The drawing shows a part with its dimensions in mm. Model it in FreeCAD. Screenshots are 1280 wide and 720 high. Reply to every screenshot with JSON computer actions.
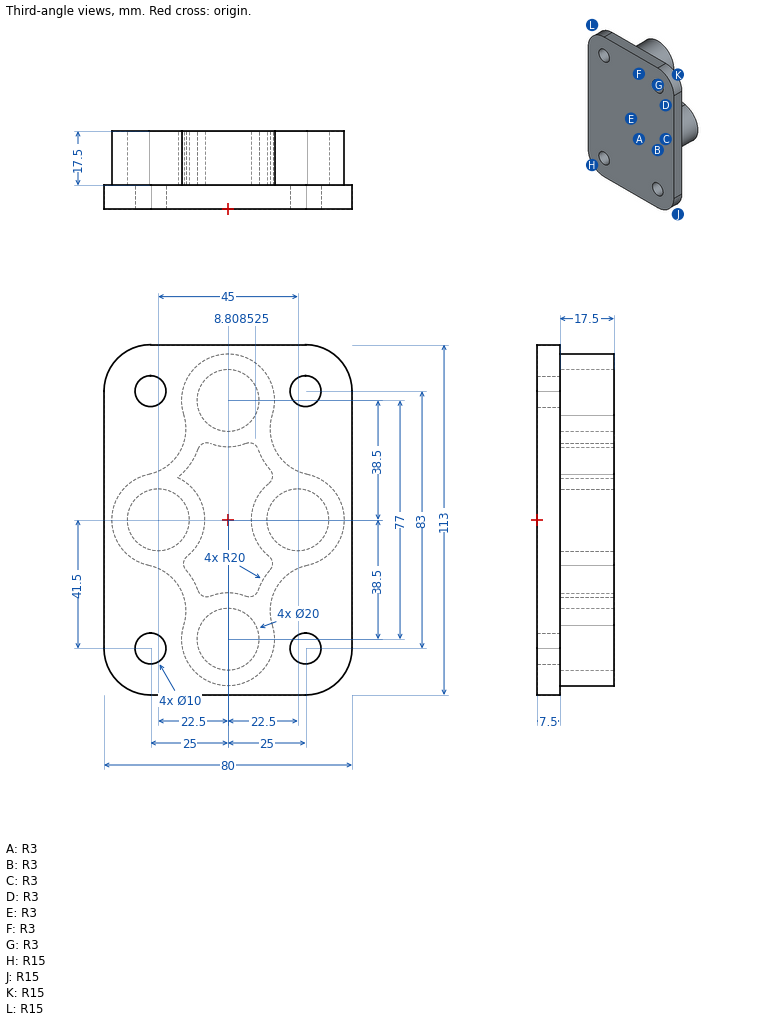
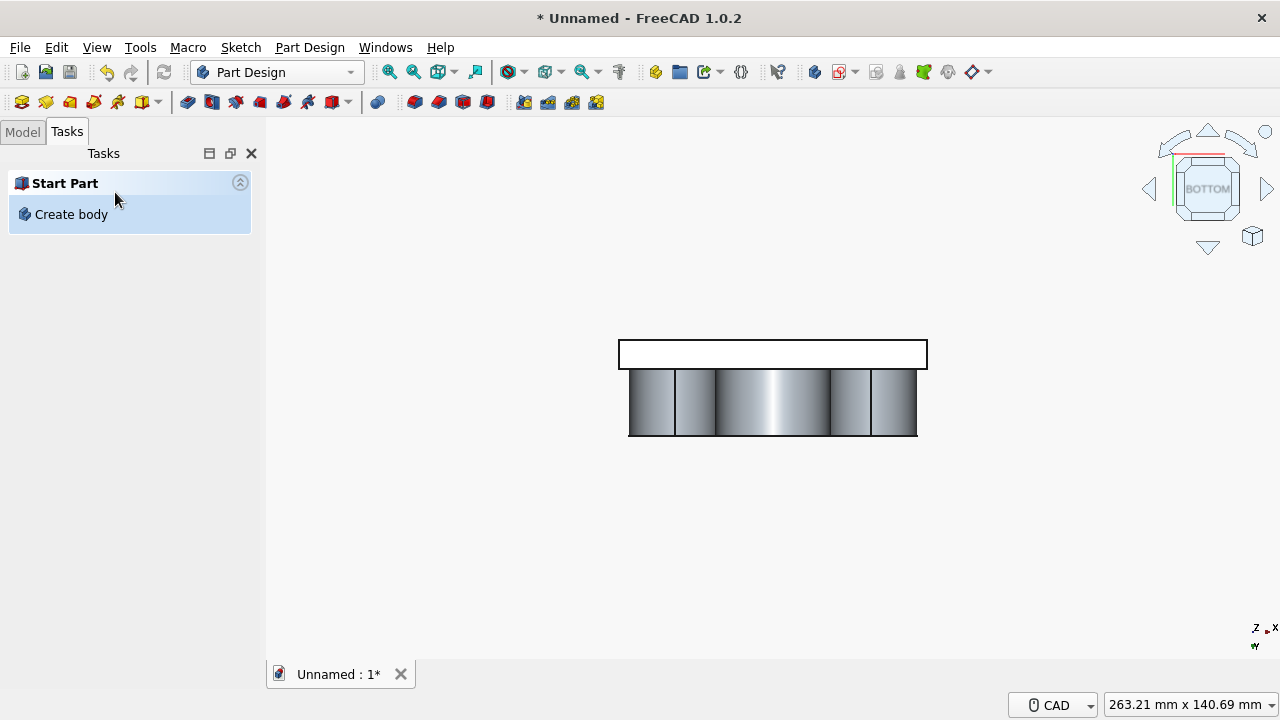
{"action": "left_click", "coordinate": [390, 72]}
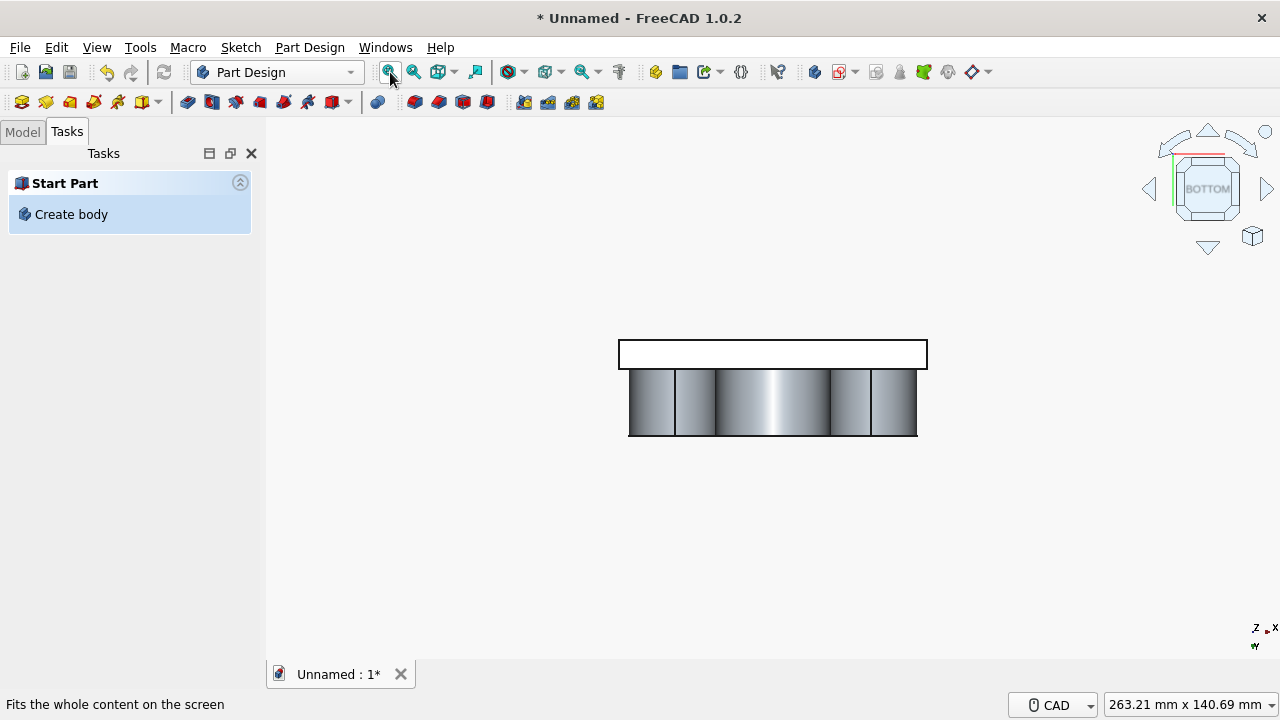
{"action": "key", "text": "4"}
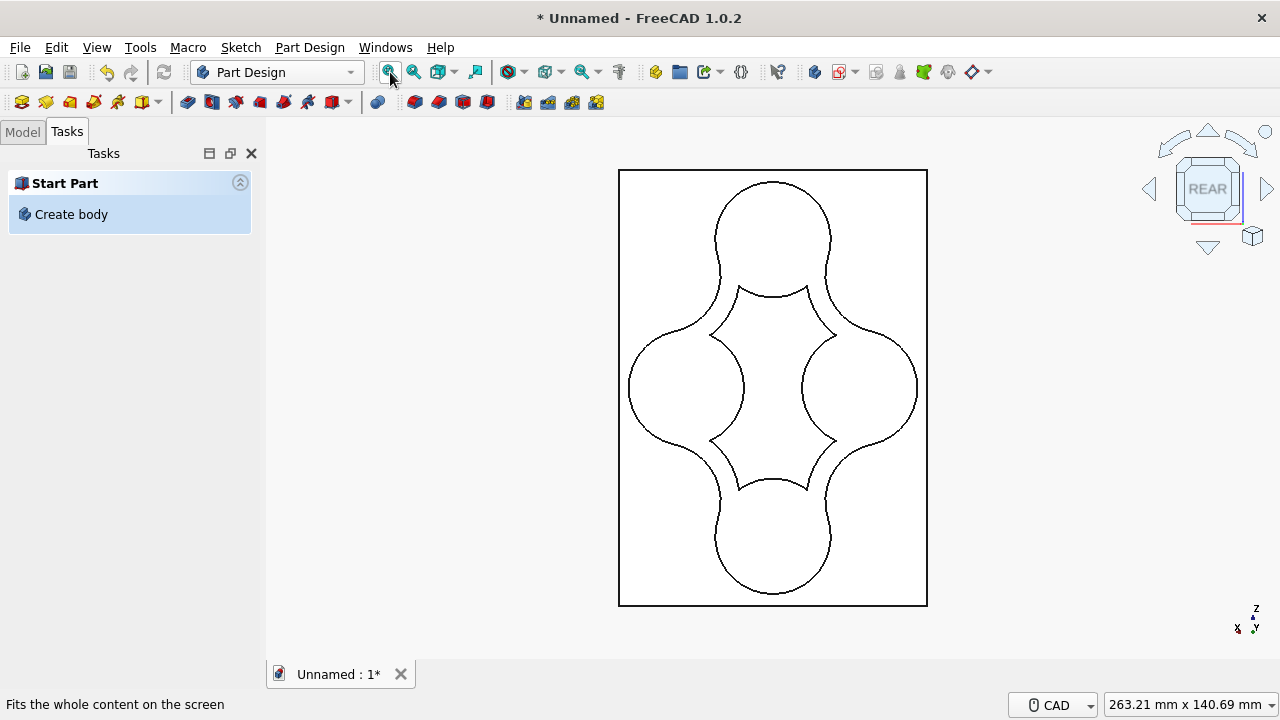
{"action": "key", "text": "6"}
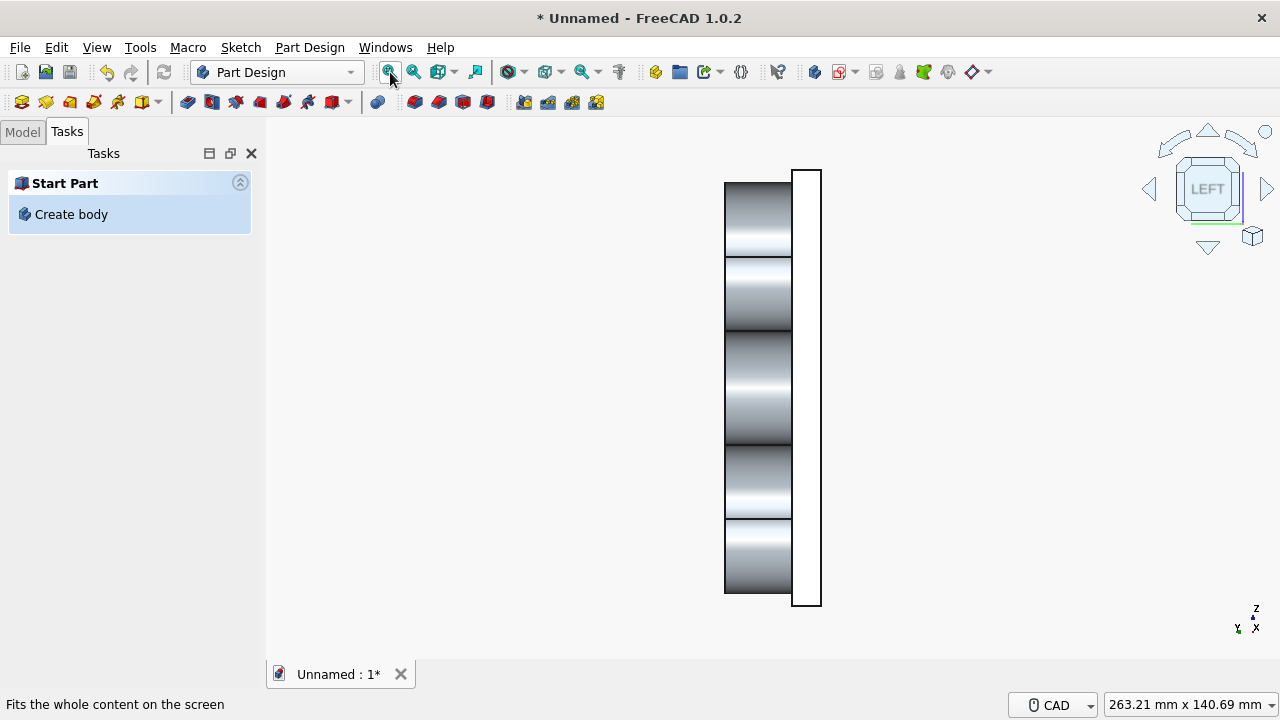
{"action": "key", "text": "v 3"}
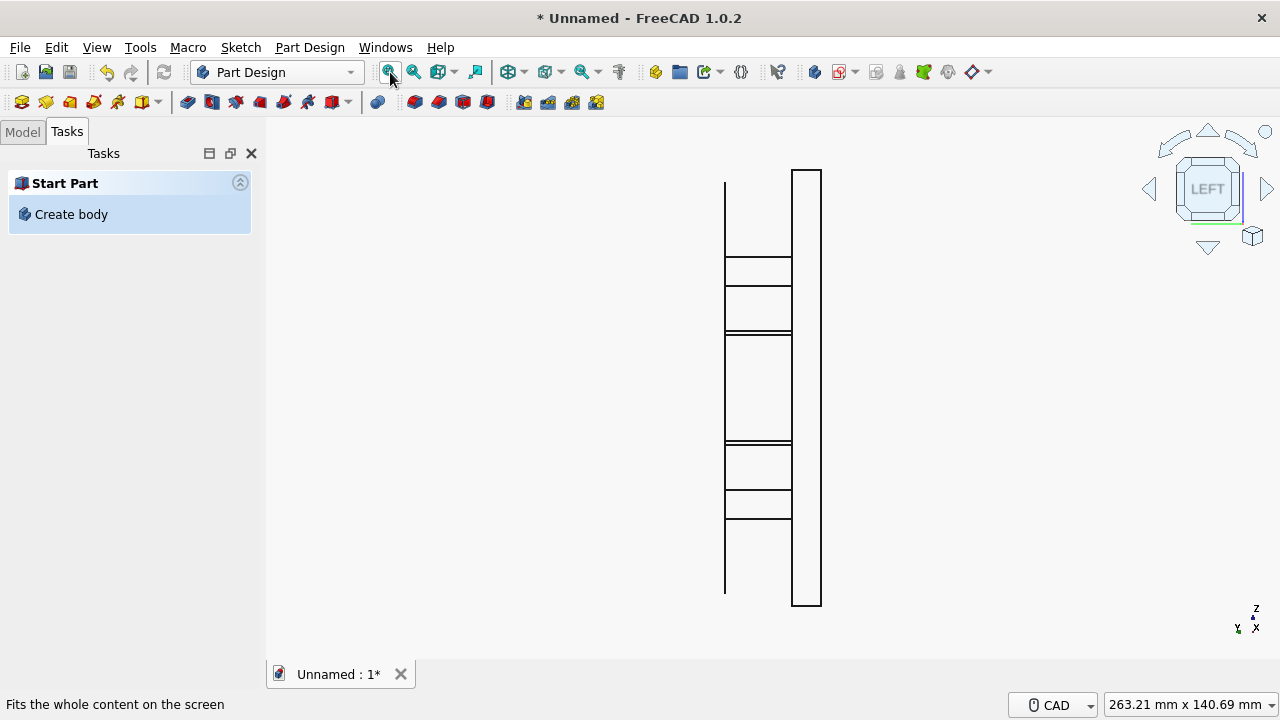
{"action": "key", "text": "0"}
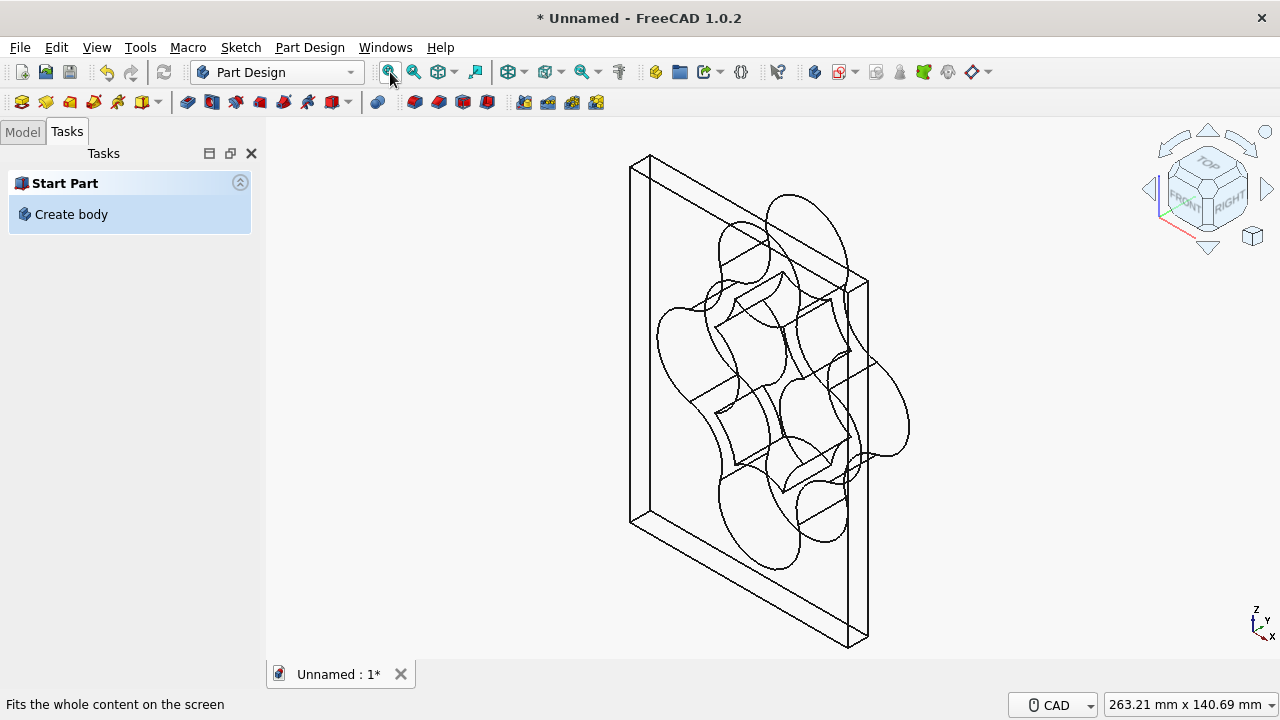
{"action": "left_click", "coordinate": [759, 450]}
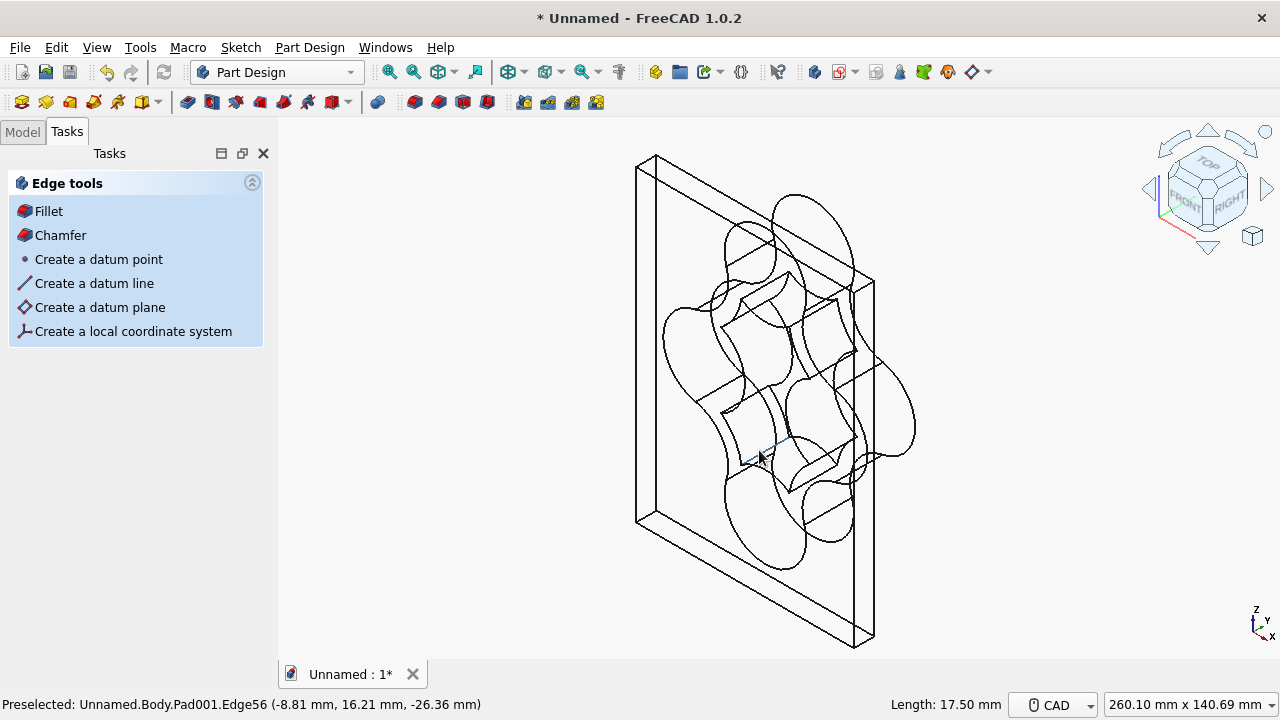
{"action": "key", "text": "v 1"}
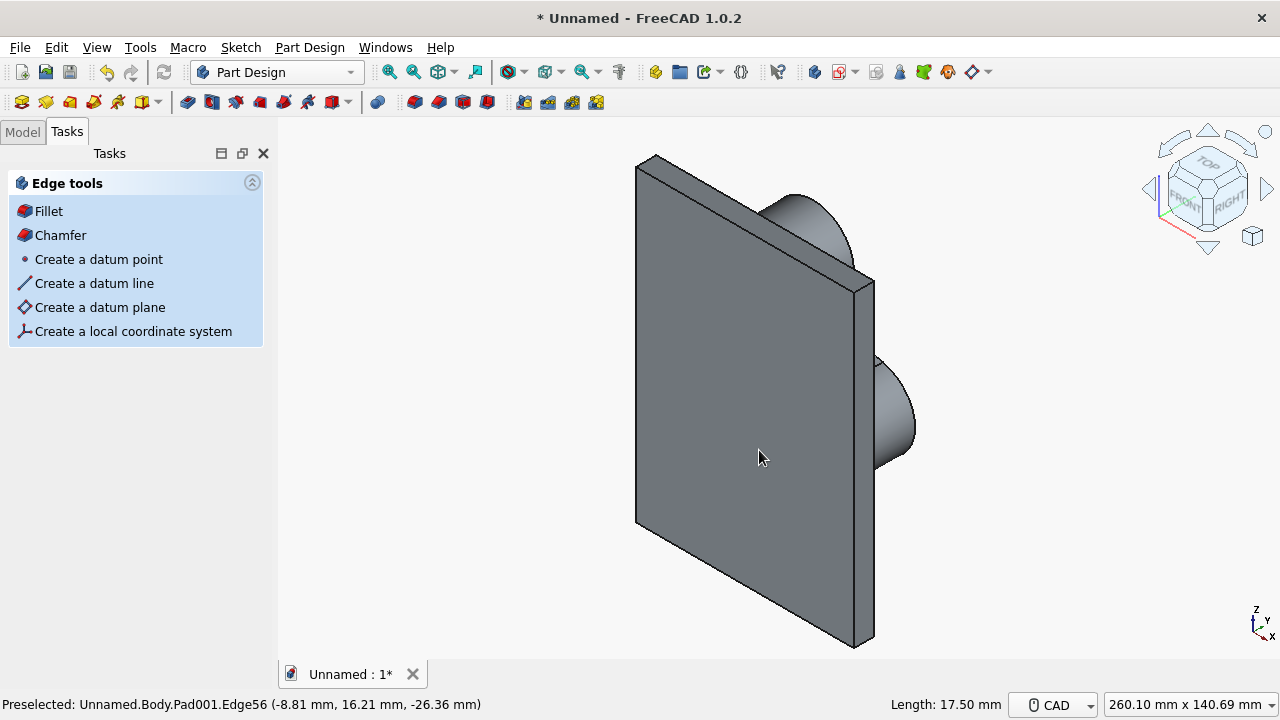
{"action": "left_click", "coordinate": [416, 102]}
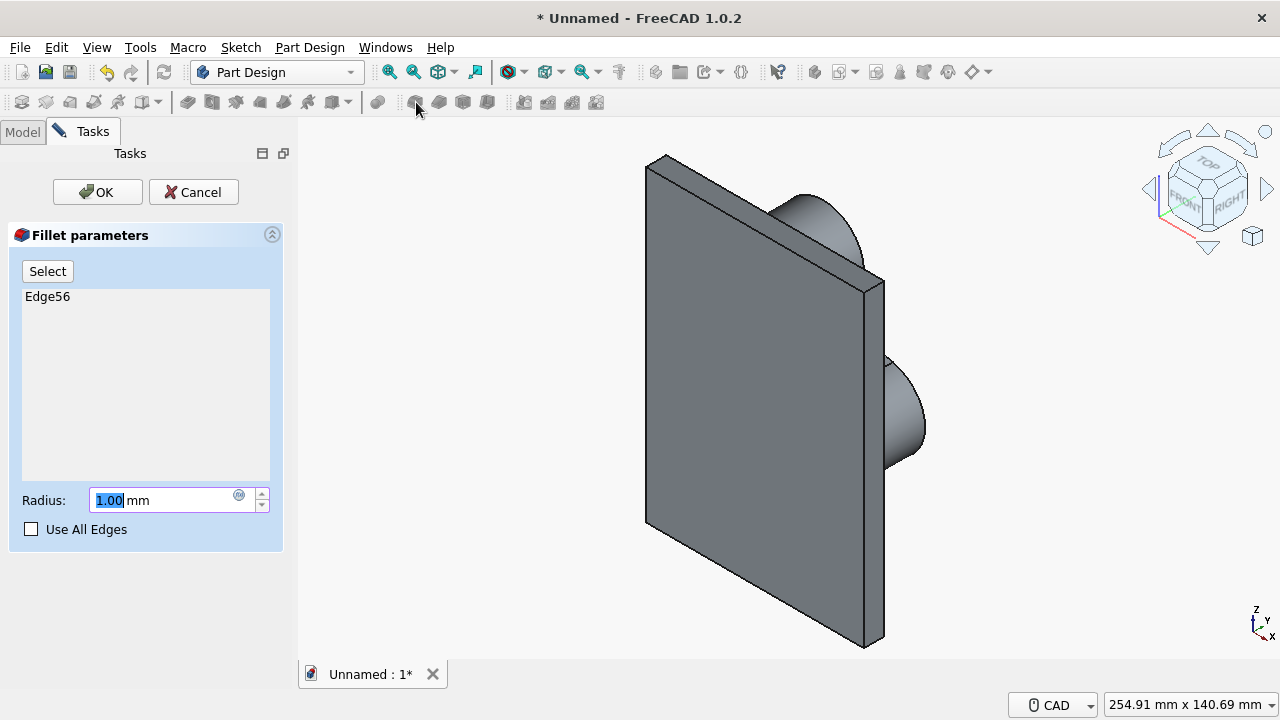
{"action": "type", "text": "3"}
{"action": "key", "text": "Tab"}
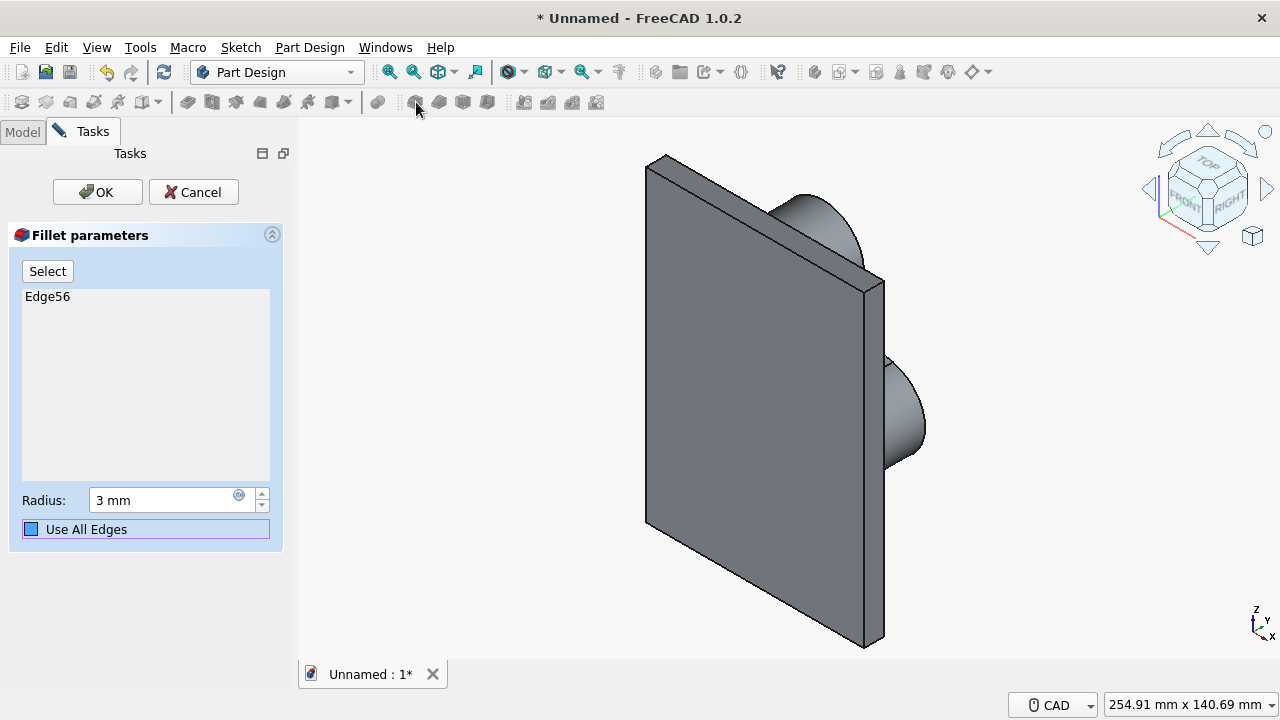
{"action": "left_click", "coordinate": [98, 192]}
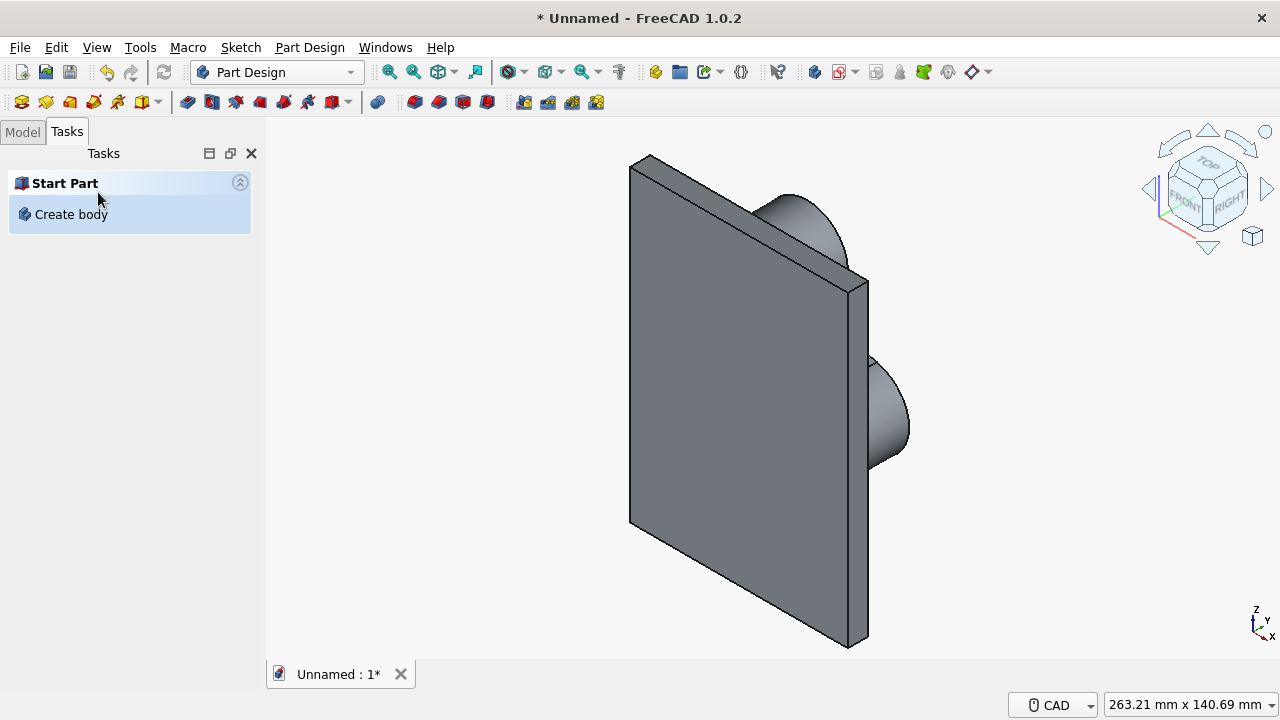
{"action": "key", "text": "2"}